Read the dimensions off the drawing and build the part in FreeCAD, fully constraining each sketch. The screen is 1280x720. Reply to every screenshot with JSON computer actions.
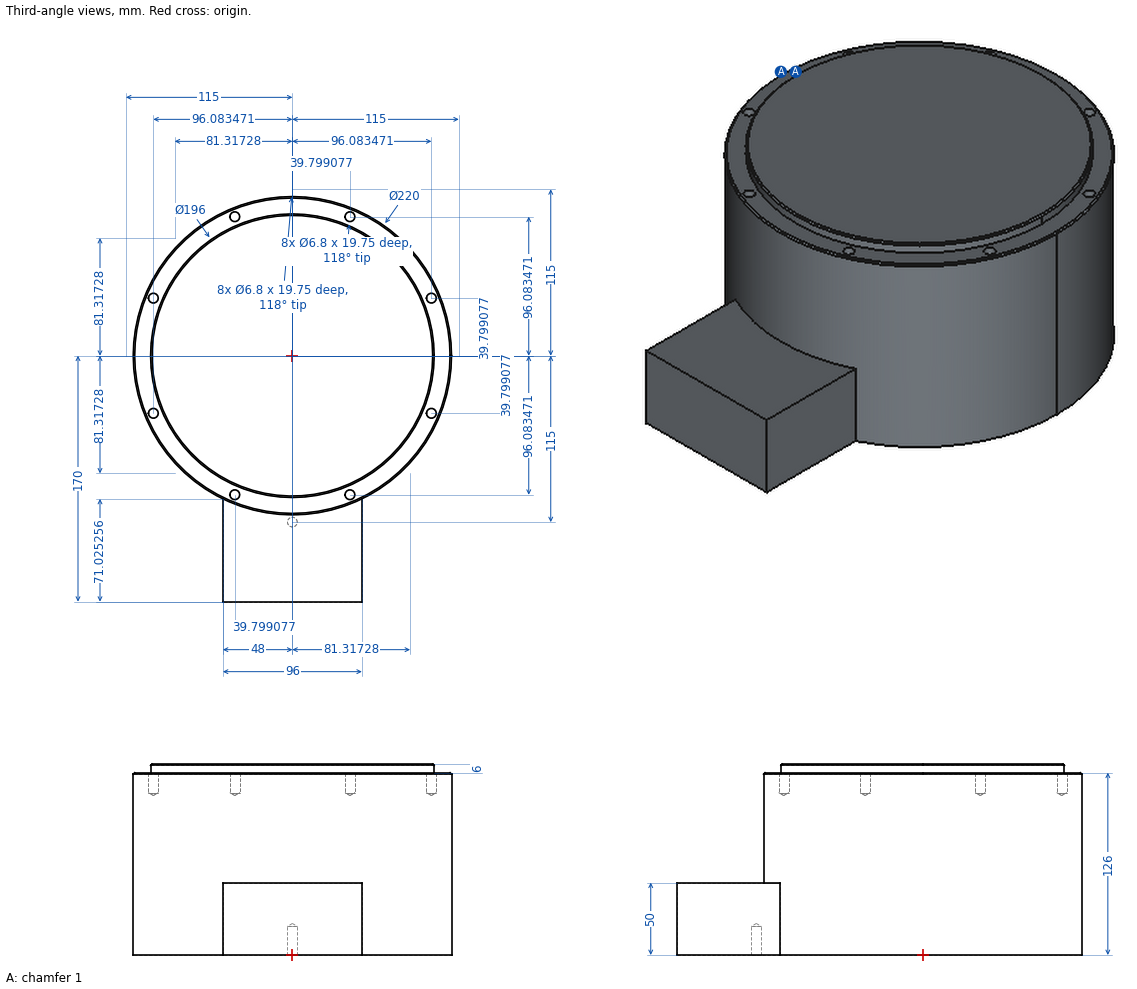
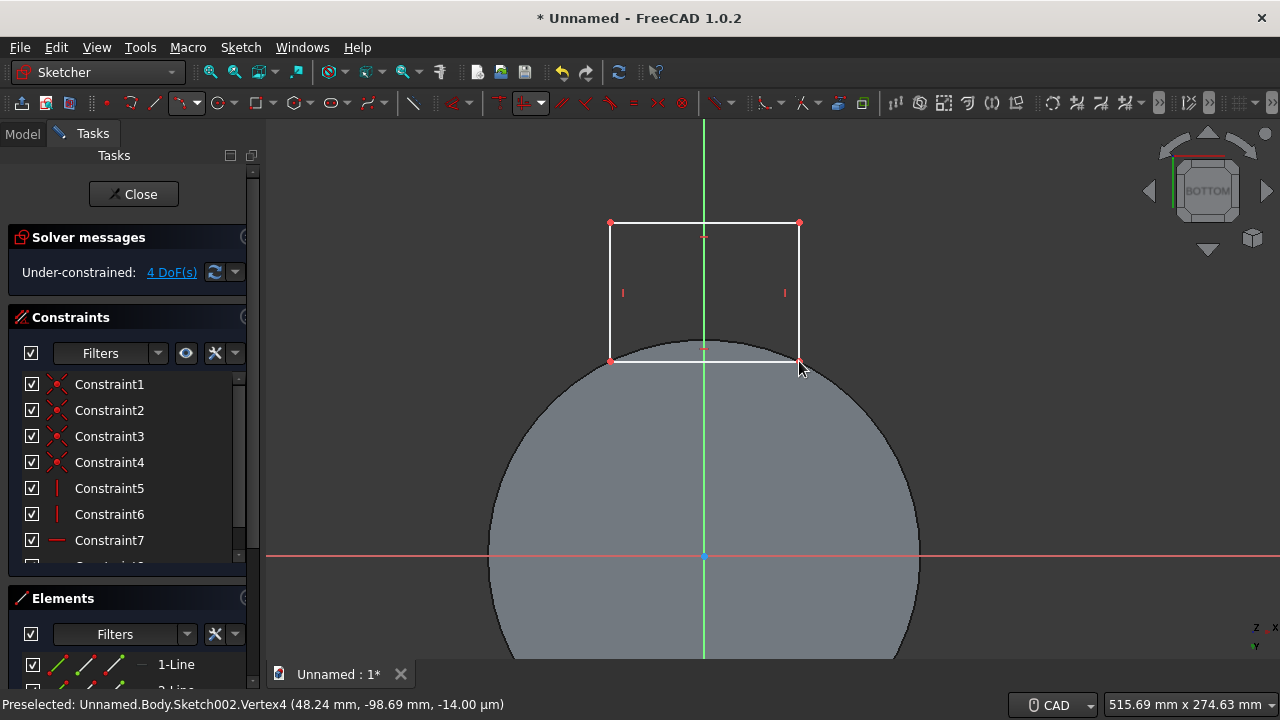
{"action": "left_click", "coordinate": [452, 104]}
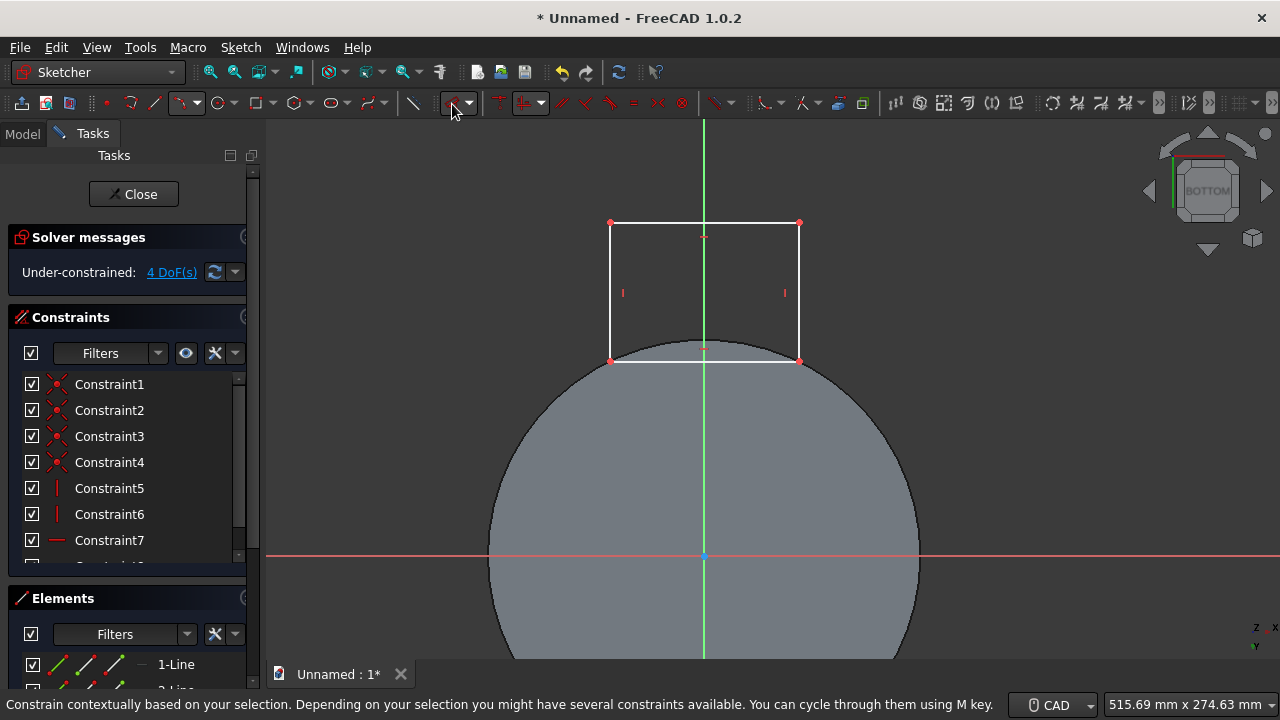
{"action": "left_click", "coordinate": [667, 362]}
{"action": "left_click", "coordinate": [661, 328]}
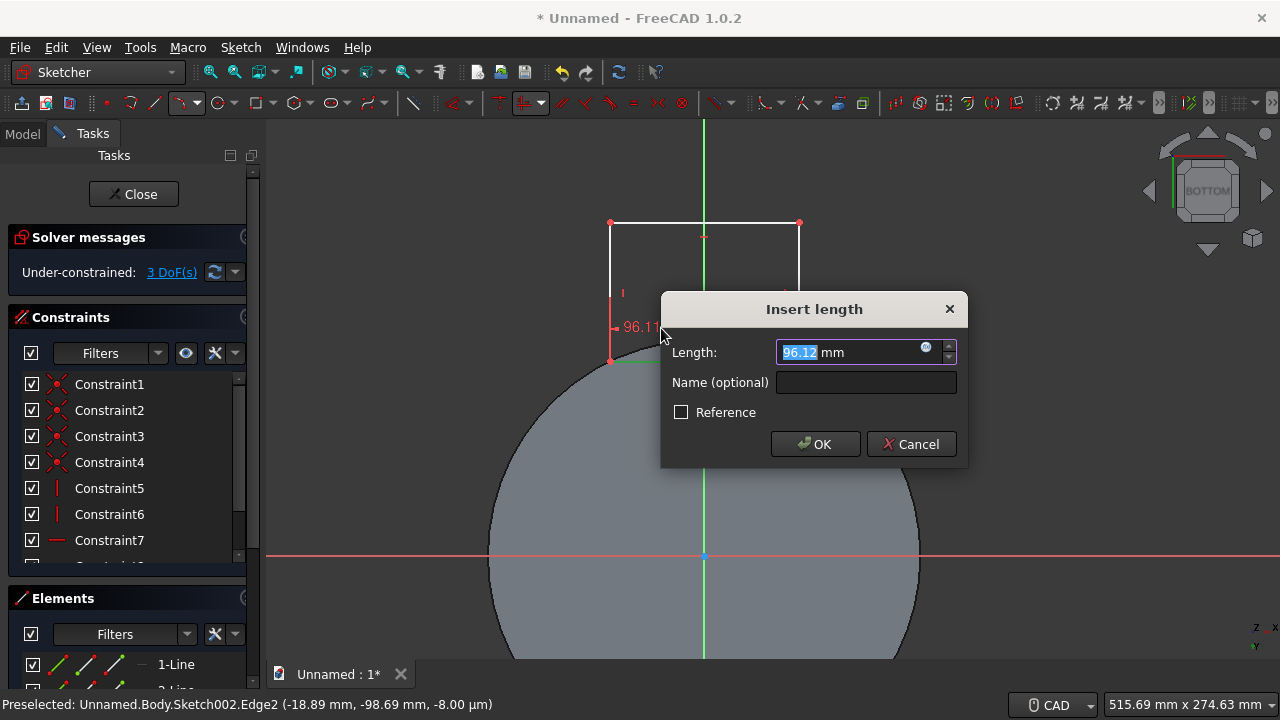
{"action": "type", "text": "96"}
{"action": "key", "text": "Return"}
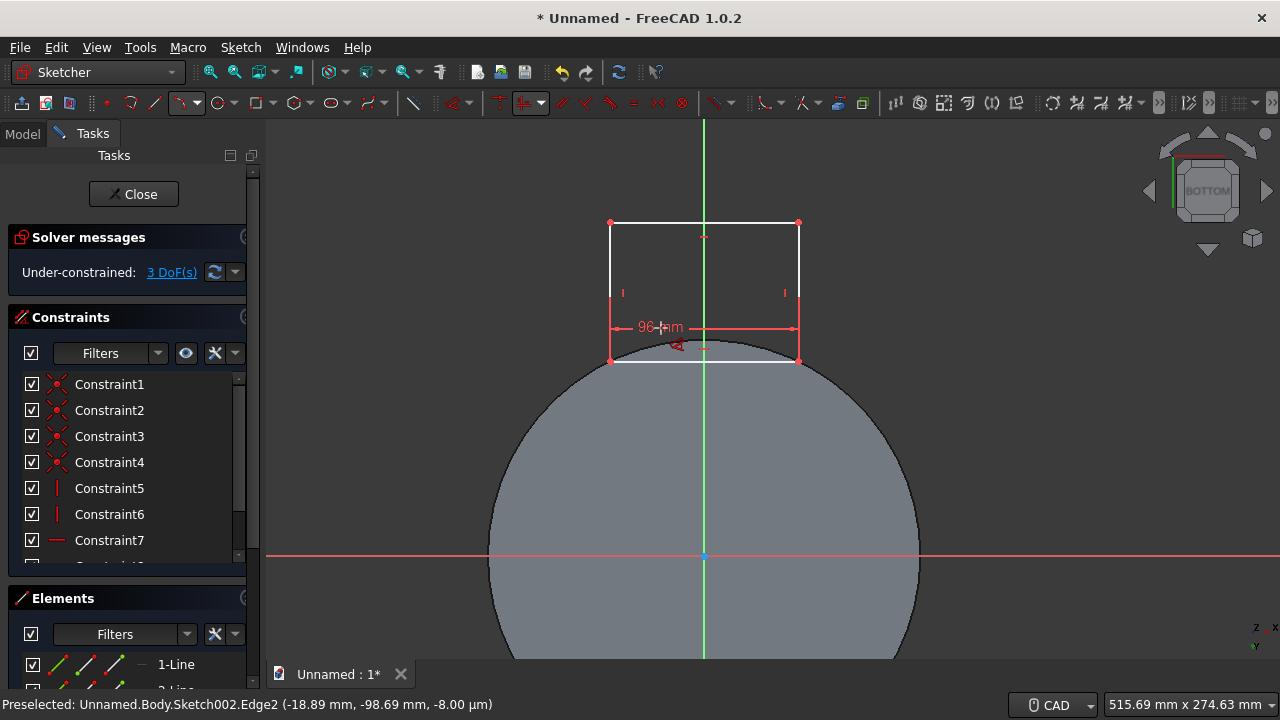
{"action": "left_click", "coordinate": [610, 223]}
{"action": "left_click", "coordinate": [657, 590]}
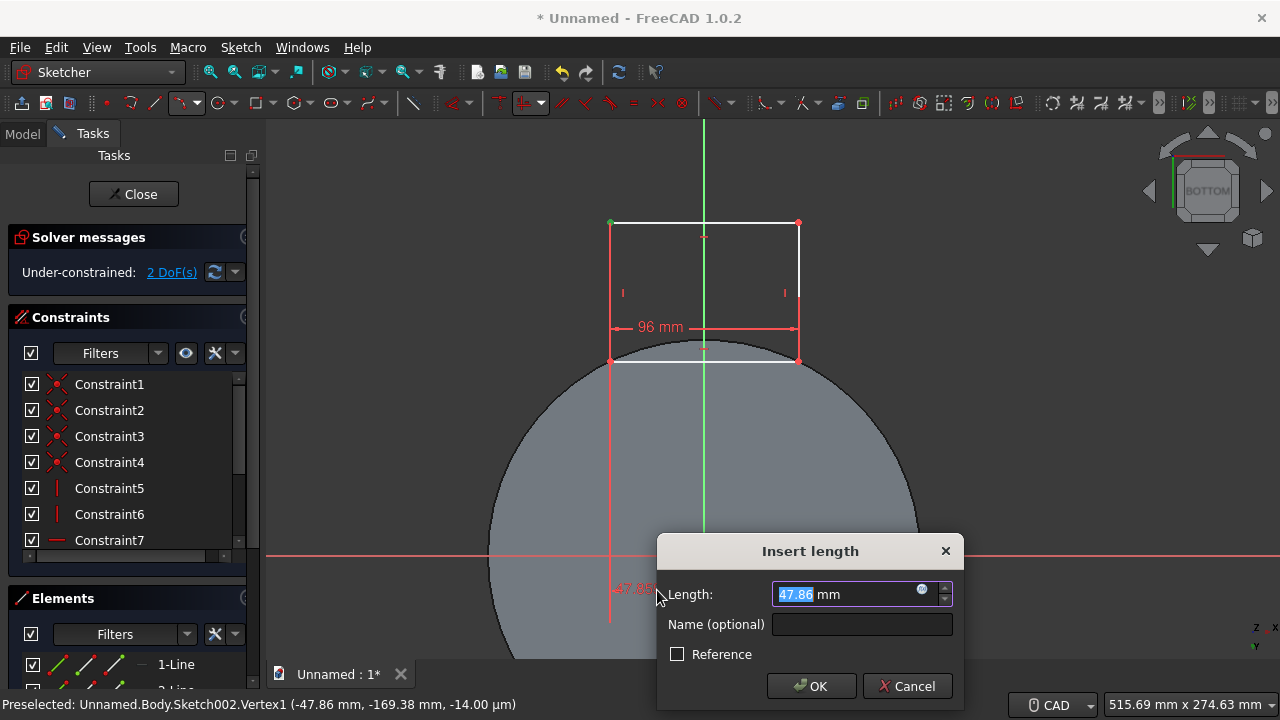
{"action": "type", "text": "48"}
{"action": "key", "text": "Return"}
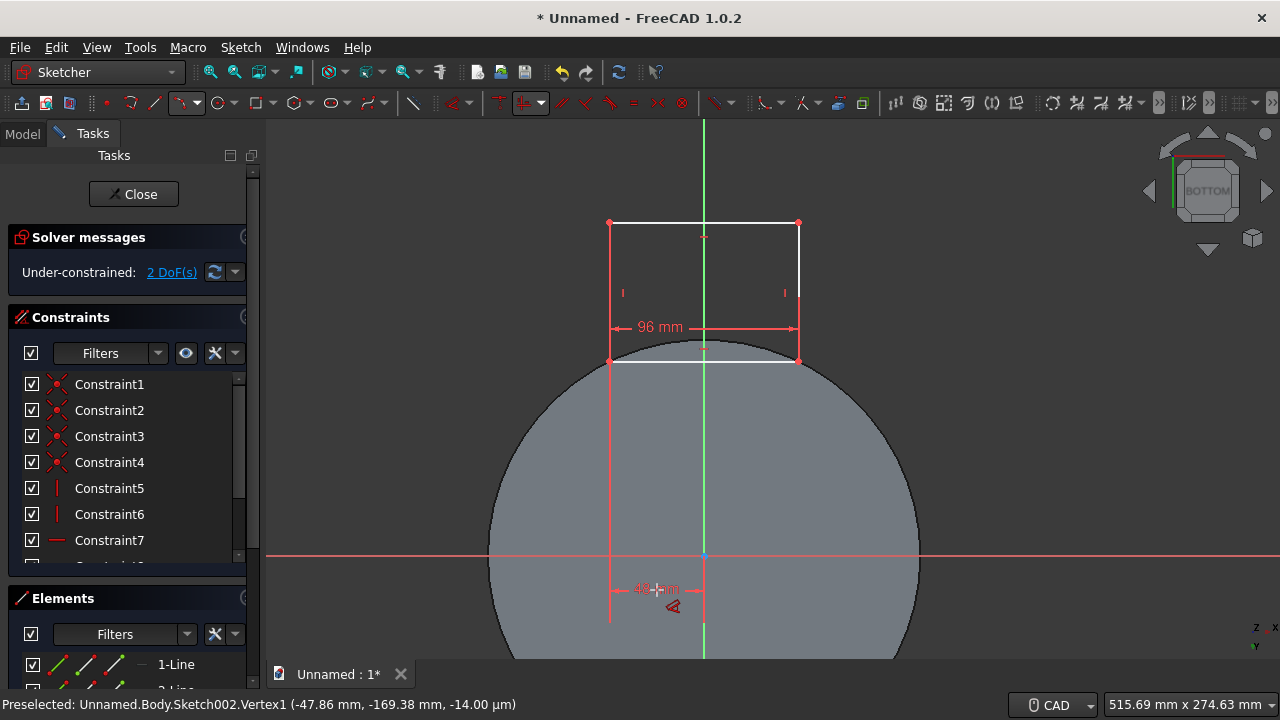
{"action": "left_click", "coordinate": [610, 223]}
{"action": "left_click", "coordinate": [576, 390]}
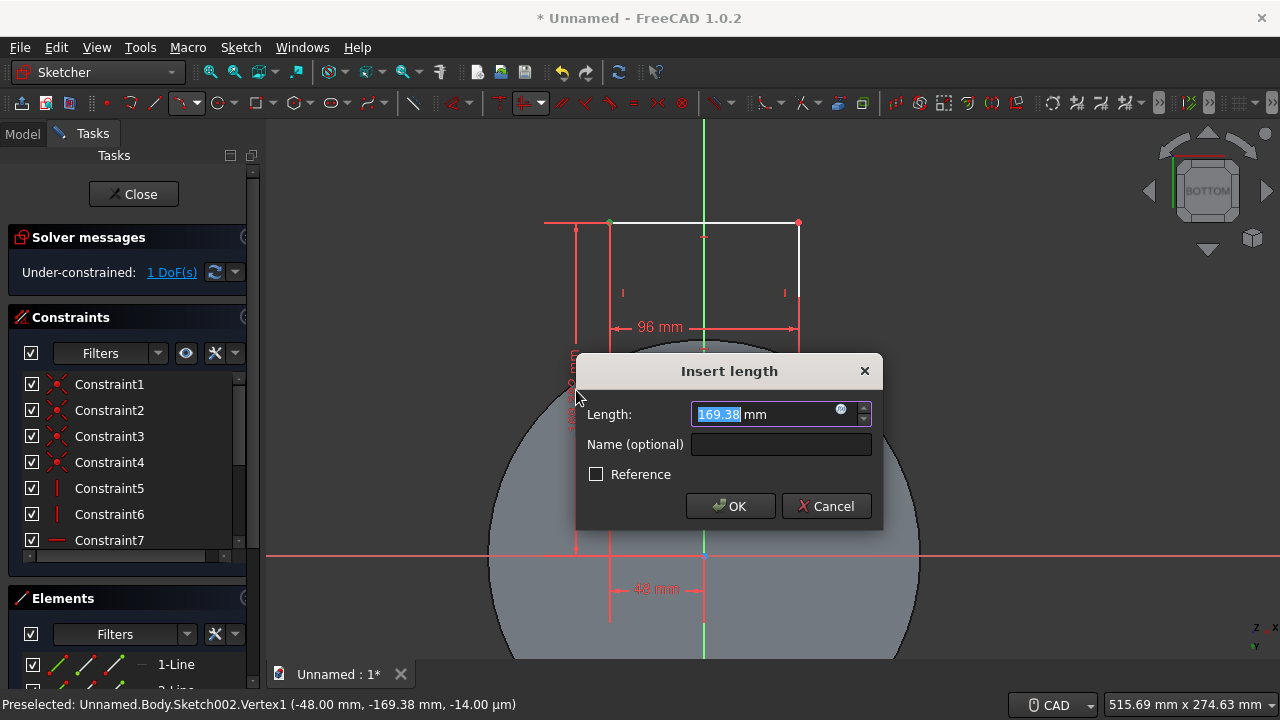
{"action": "type", "text": "170"}
{"action": "key", "text": "Return"}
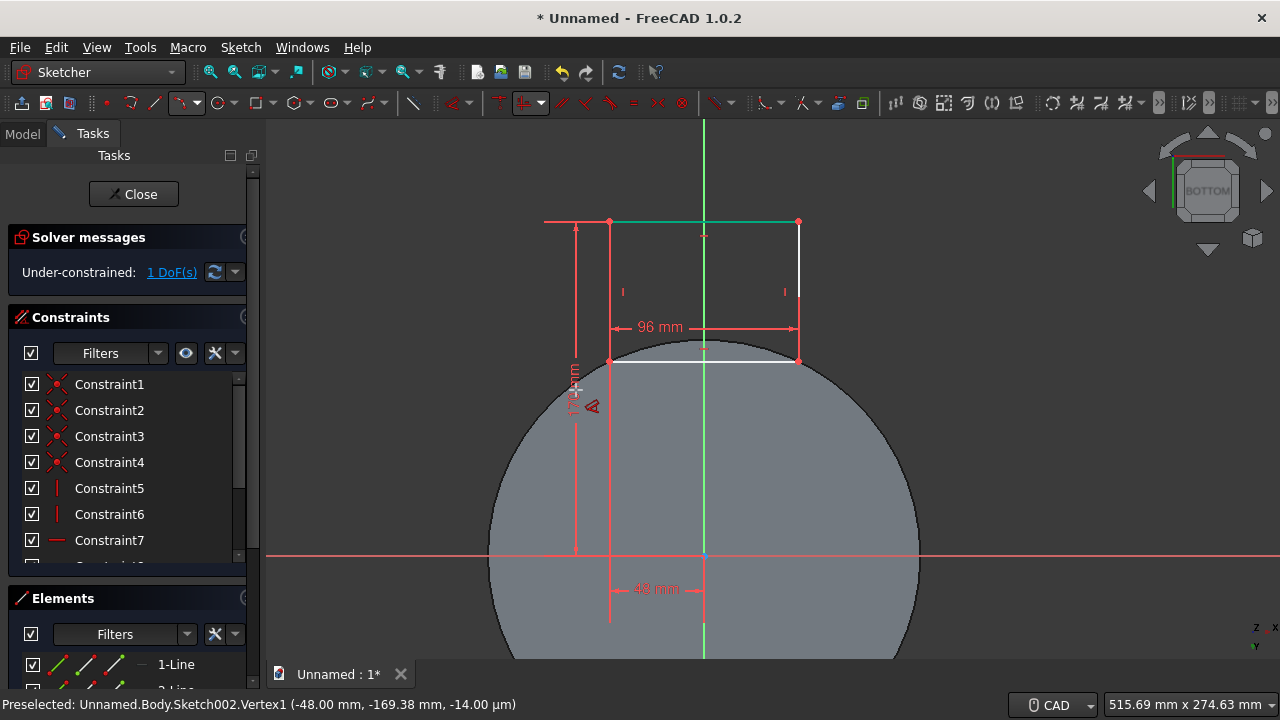
{"action": "left_click", "coordinate": [610, 264]}
{"action": "left_click", "coordinate": [576, 292]}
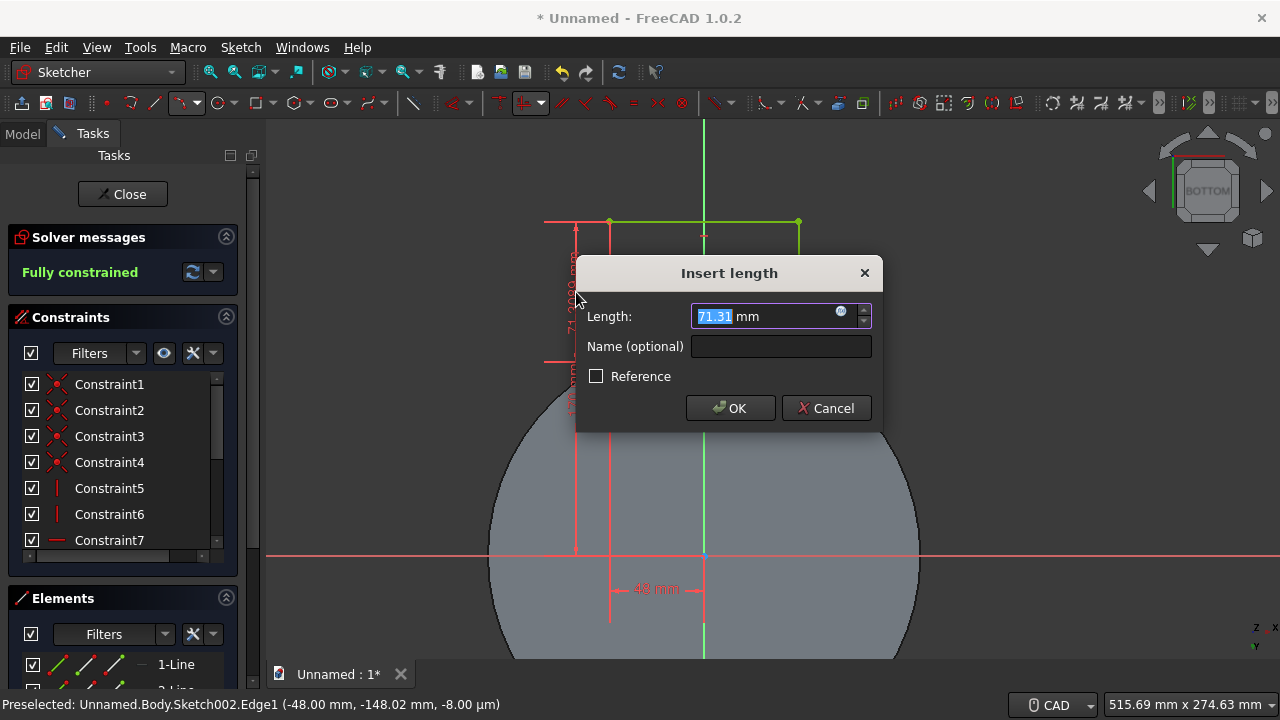
{"action": "type", "text": "71.025256"}
{"action": "key", "text": "Return"}
{"action": "key", "text": "Escape"}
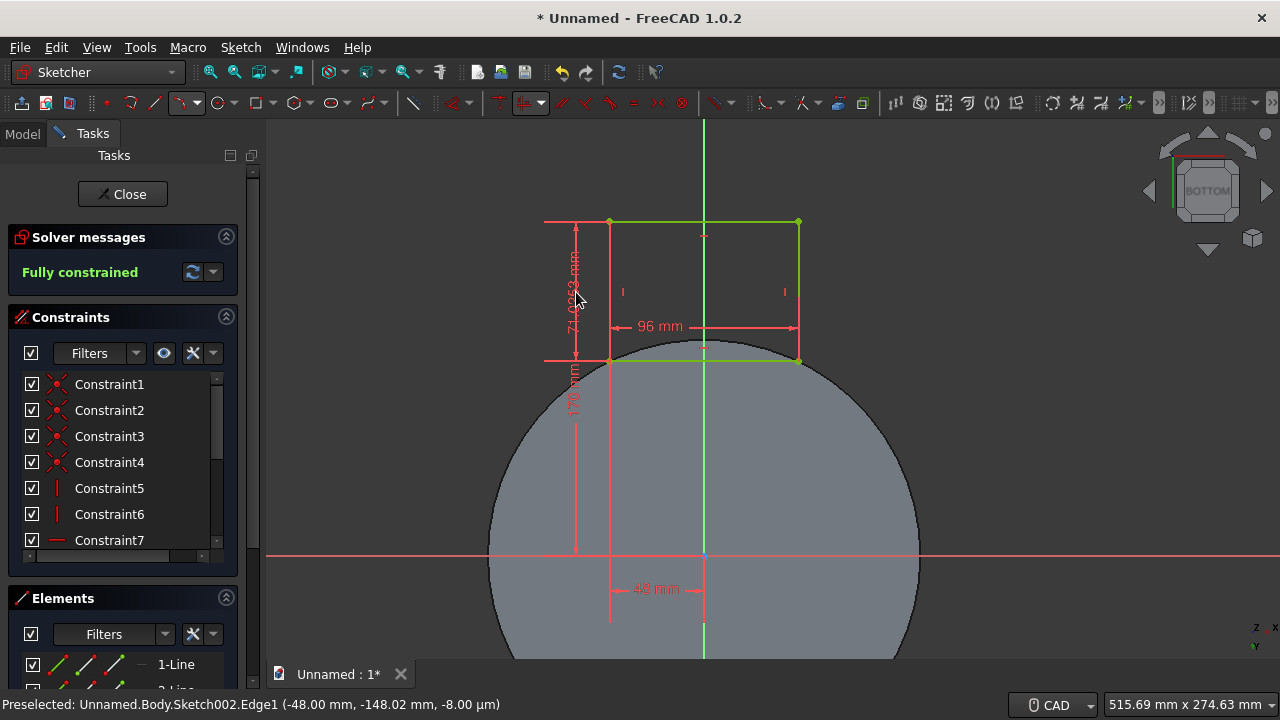
{"action": "left_click", "coordinate": [123, 194]}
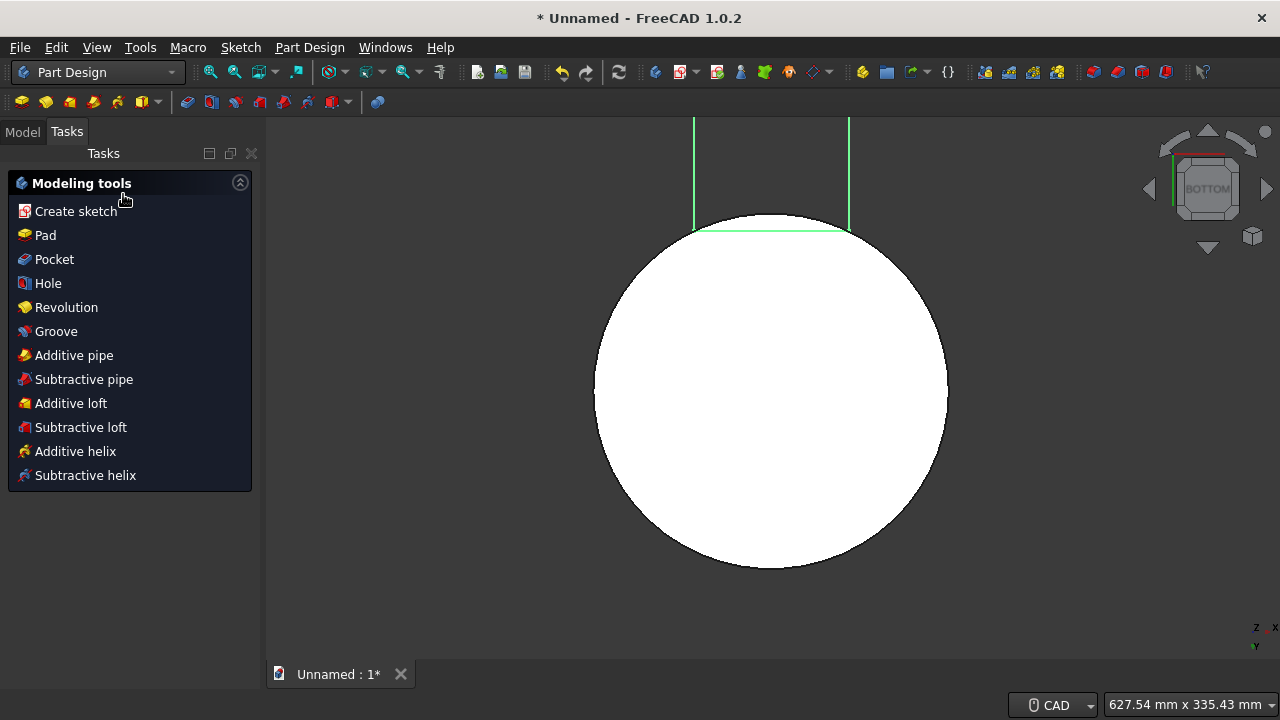
{"action": "left_click", "coordinate": [22, 102]}